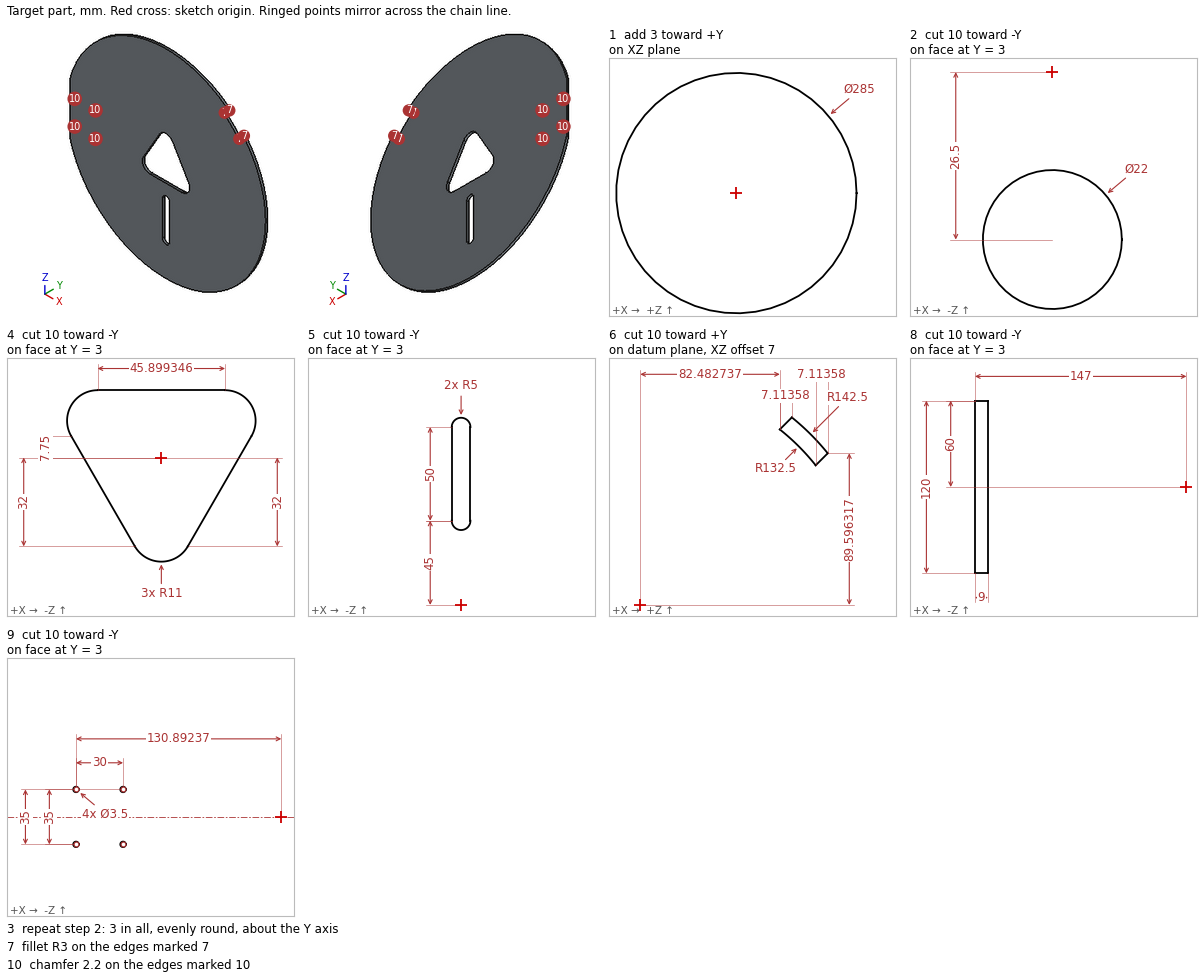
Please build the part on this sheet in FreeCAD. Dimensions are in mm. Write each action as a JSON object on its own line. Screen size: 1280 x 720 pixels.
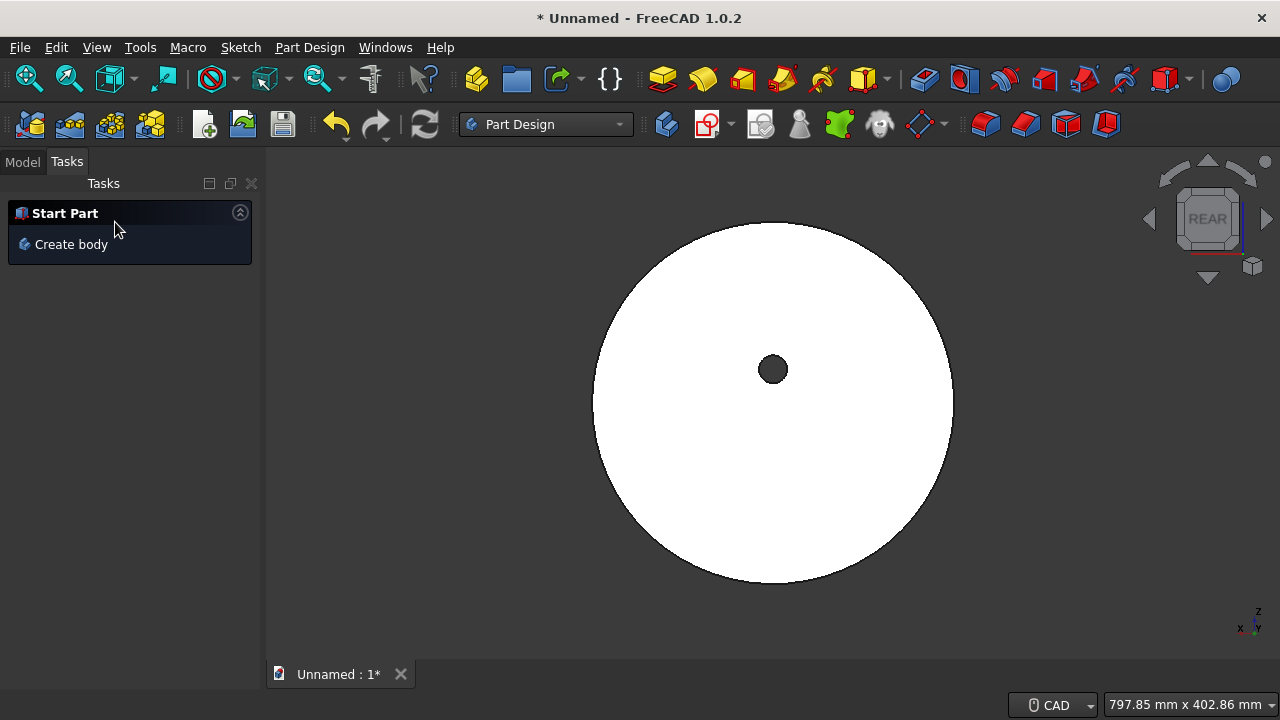
{"action": "left_click", "coordinate": [23, 161]}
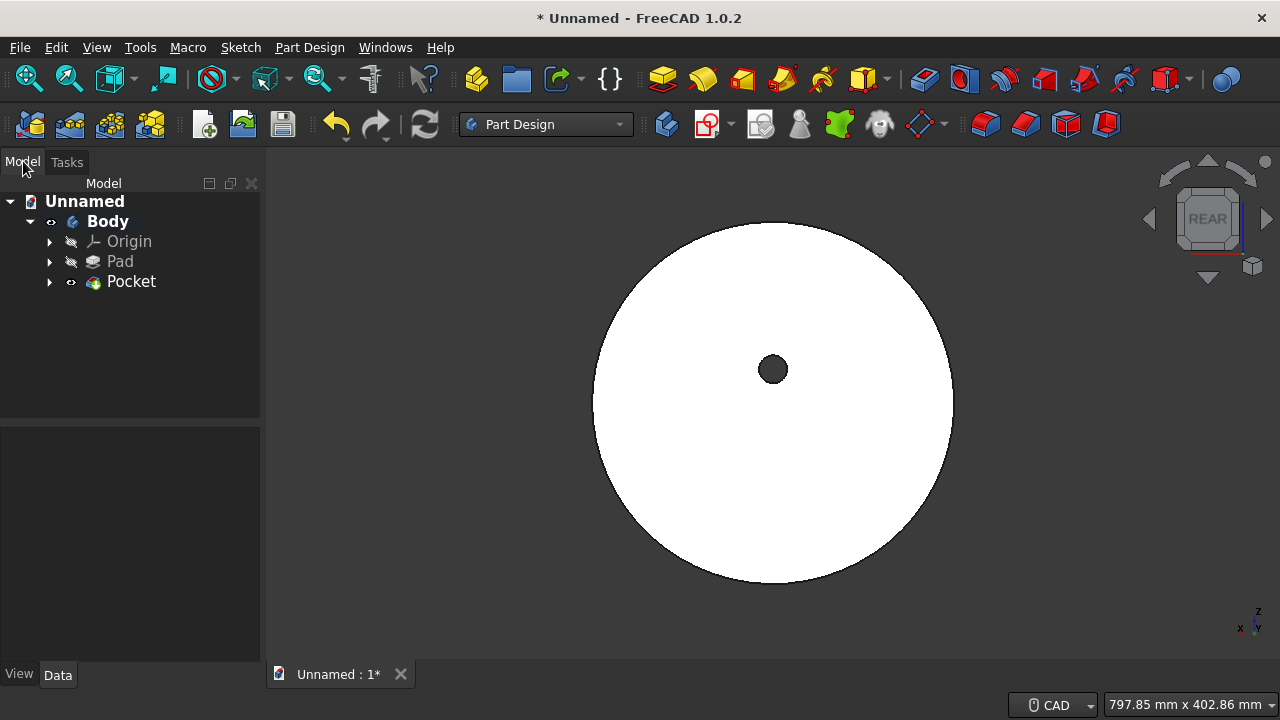
{"action": "left_click", "coordinate": [116, 282]}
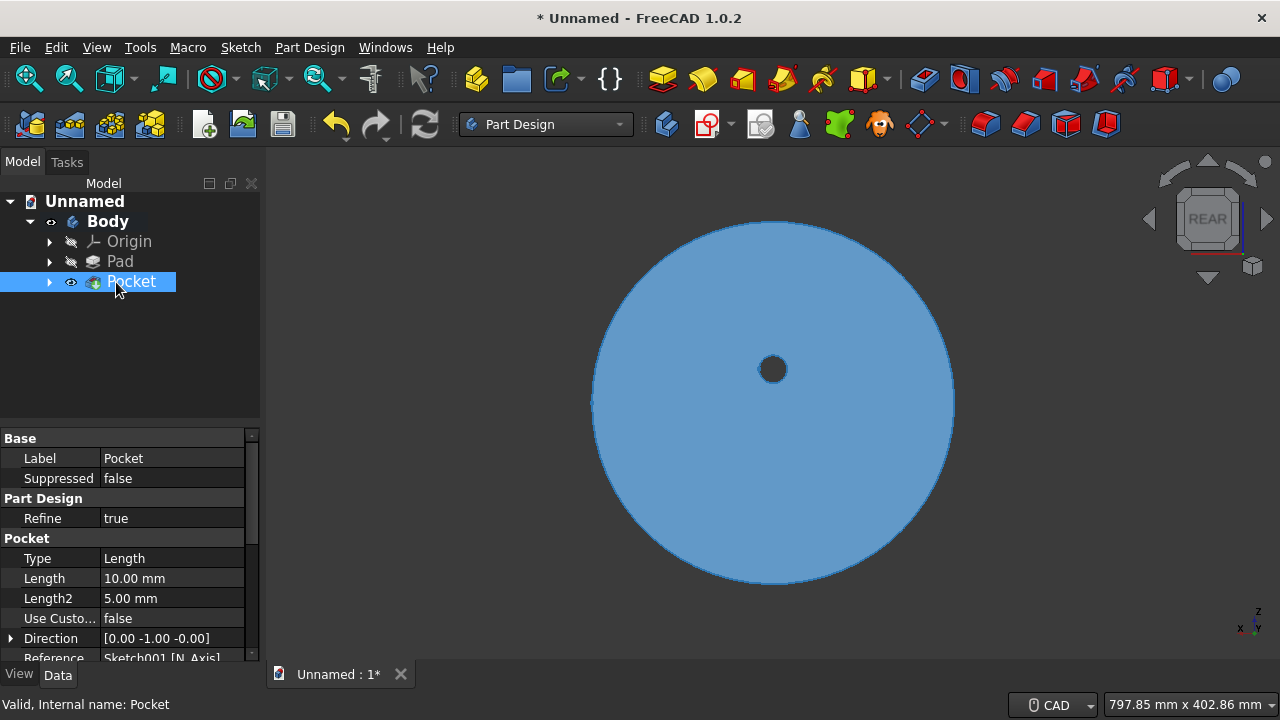
{"action": "left_click", "coordinate": [110, 124]}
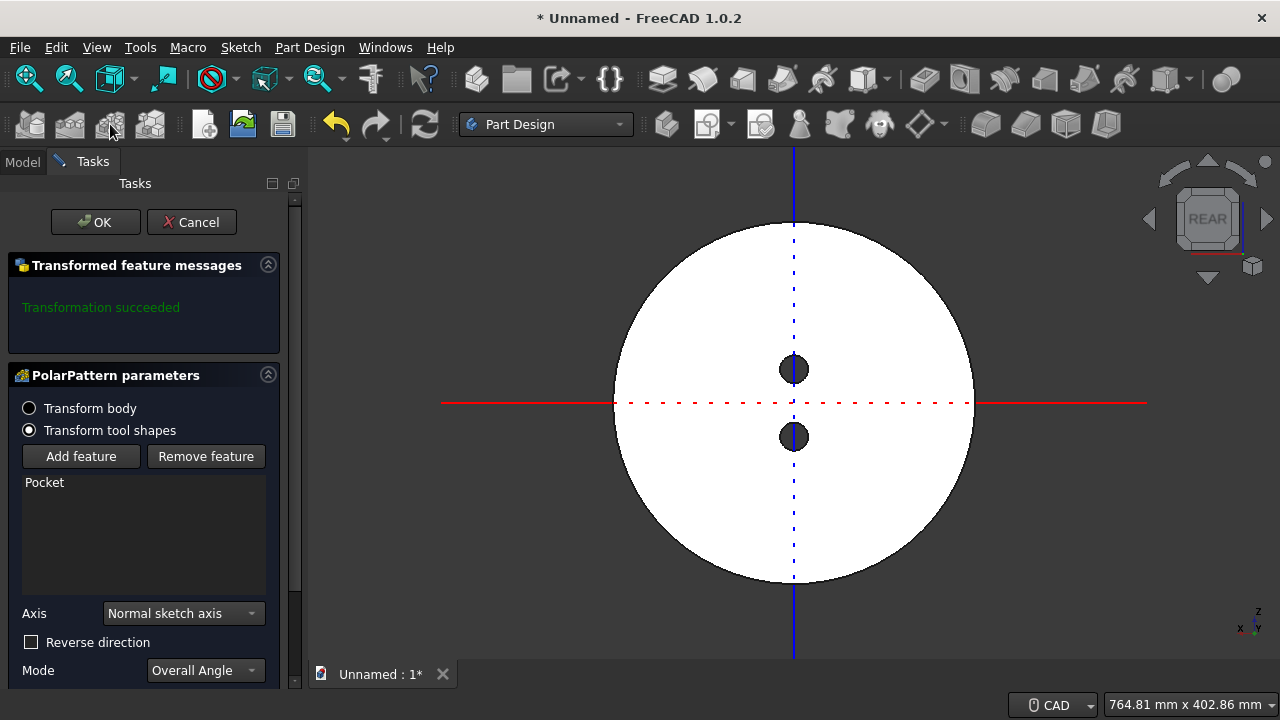
{"action": "left_click", "coordinate": [184, 614]}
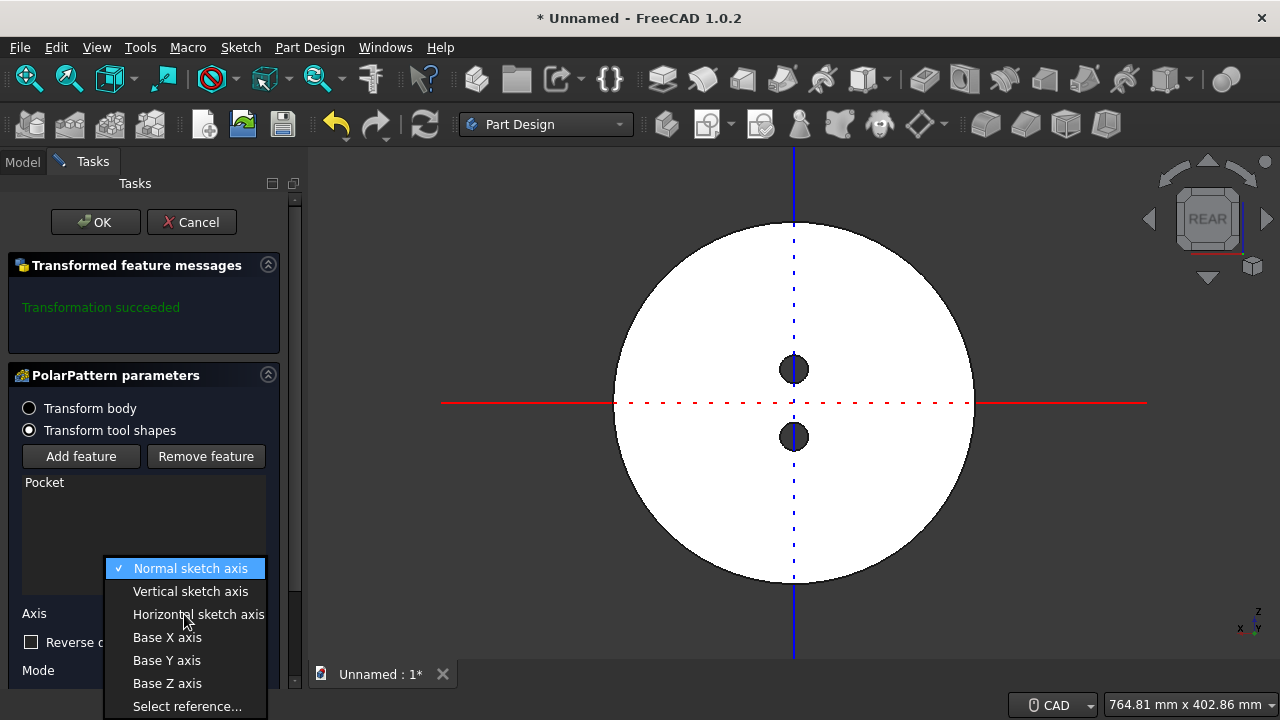
{"action": "left_click", "coordinate": [184, 660]}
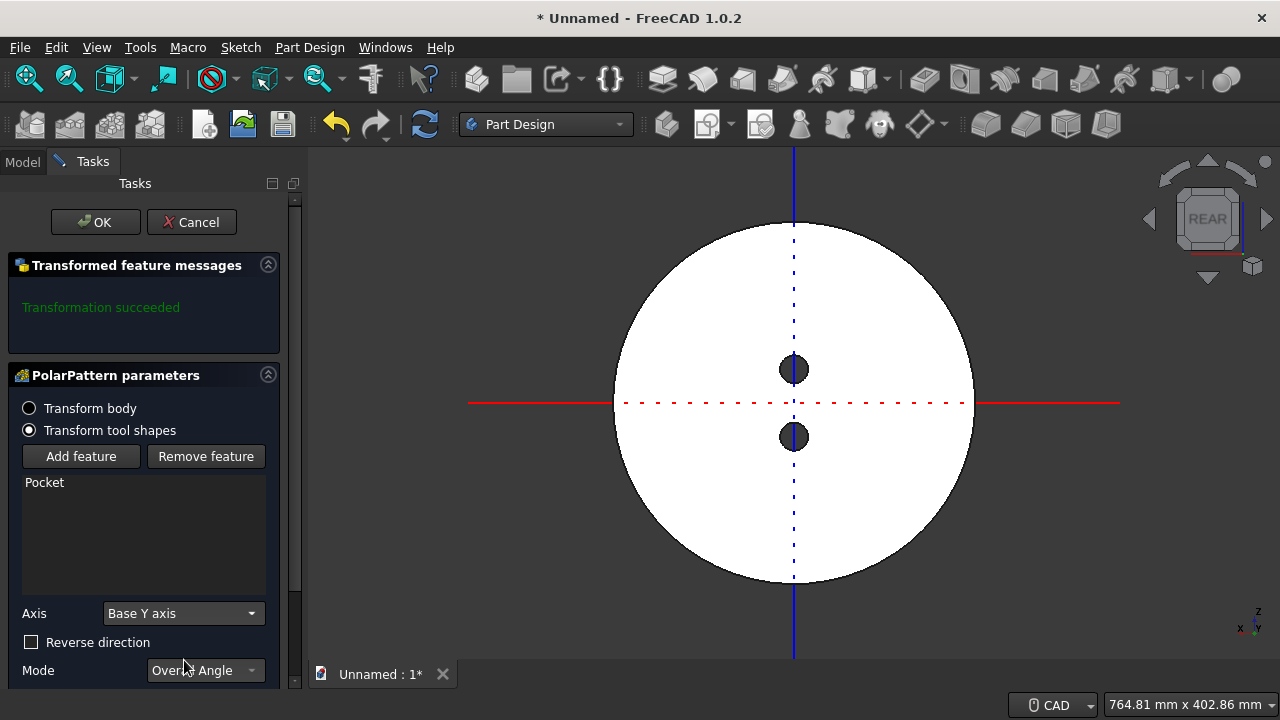
{"action": "scroll", "coordinate": [295, 440], "scroll_direction": "down", "scroll_amount": 2}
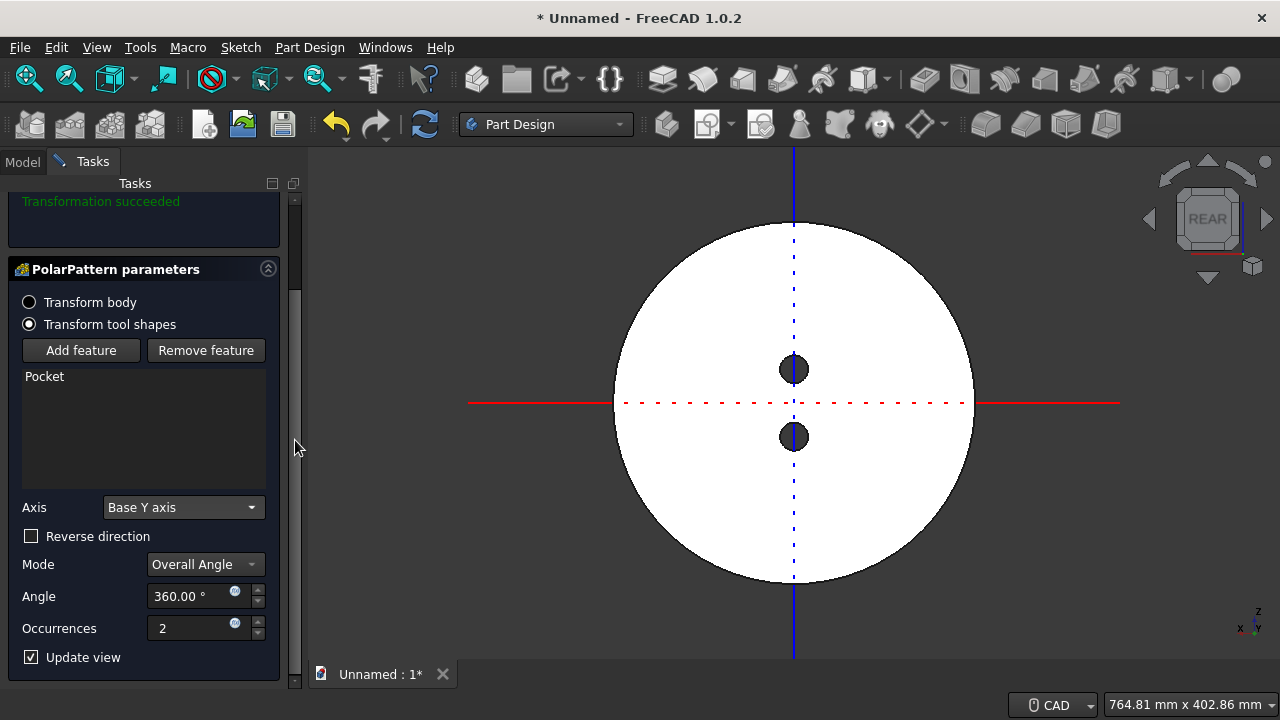
{"action": "triple_click", "coordinate": [198, 628]}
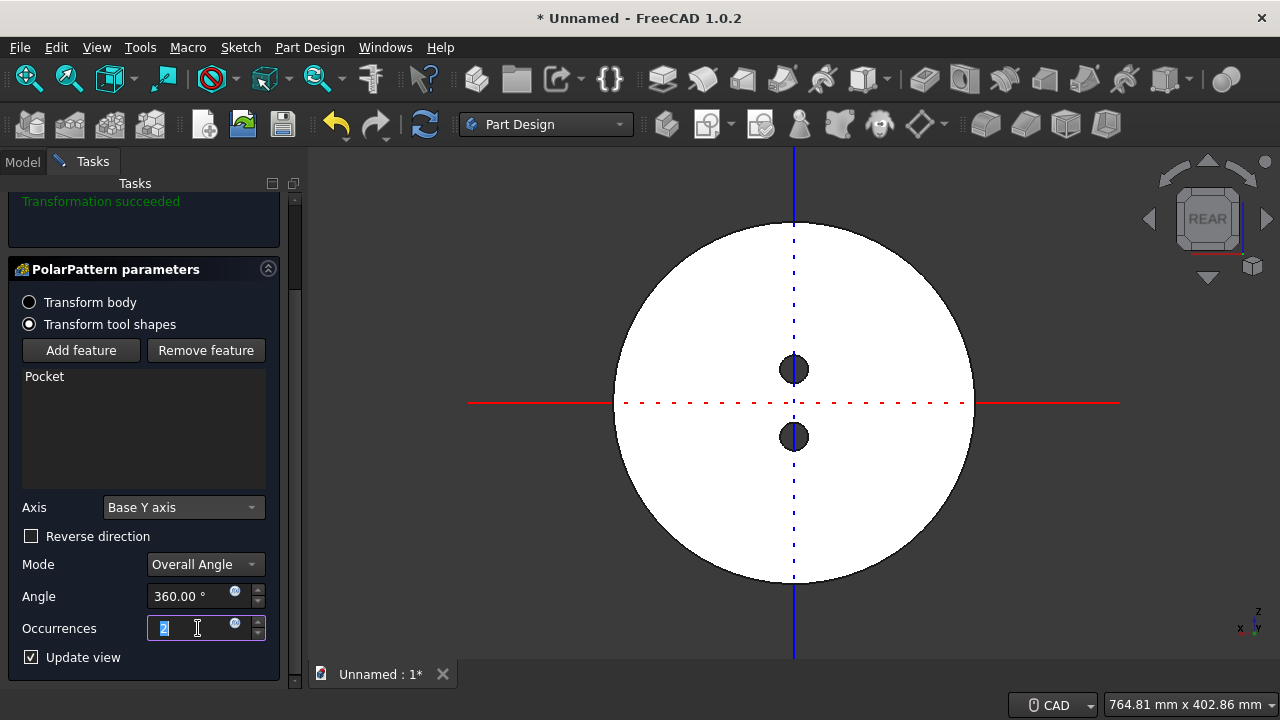
{"action": "type", "text": "3"}
{"action": "key", "text": "Tab"}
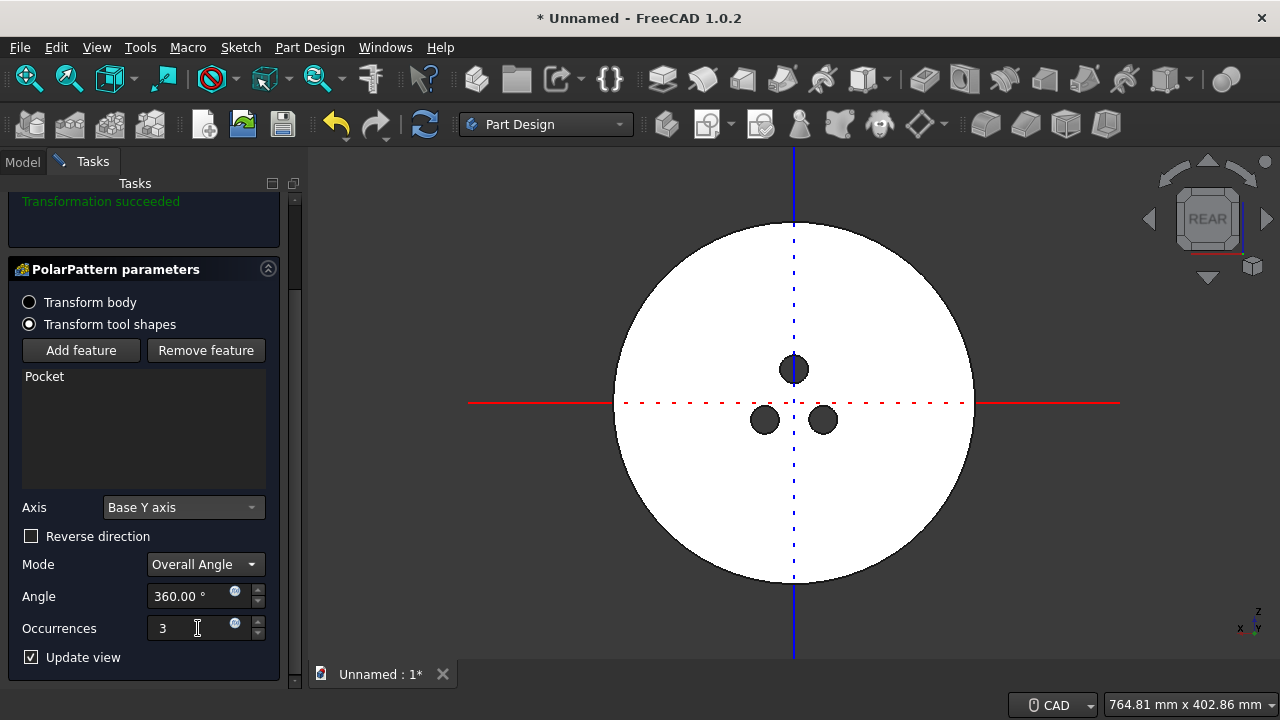
{"action": "scroll", "coordinate": [295, 440], "scroll_direction": "up", "scroll_amount": 3}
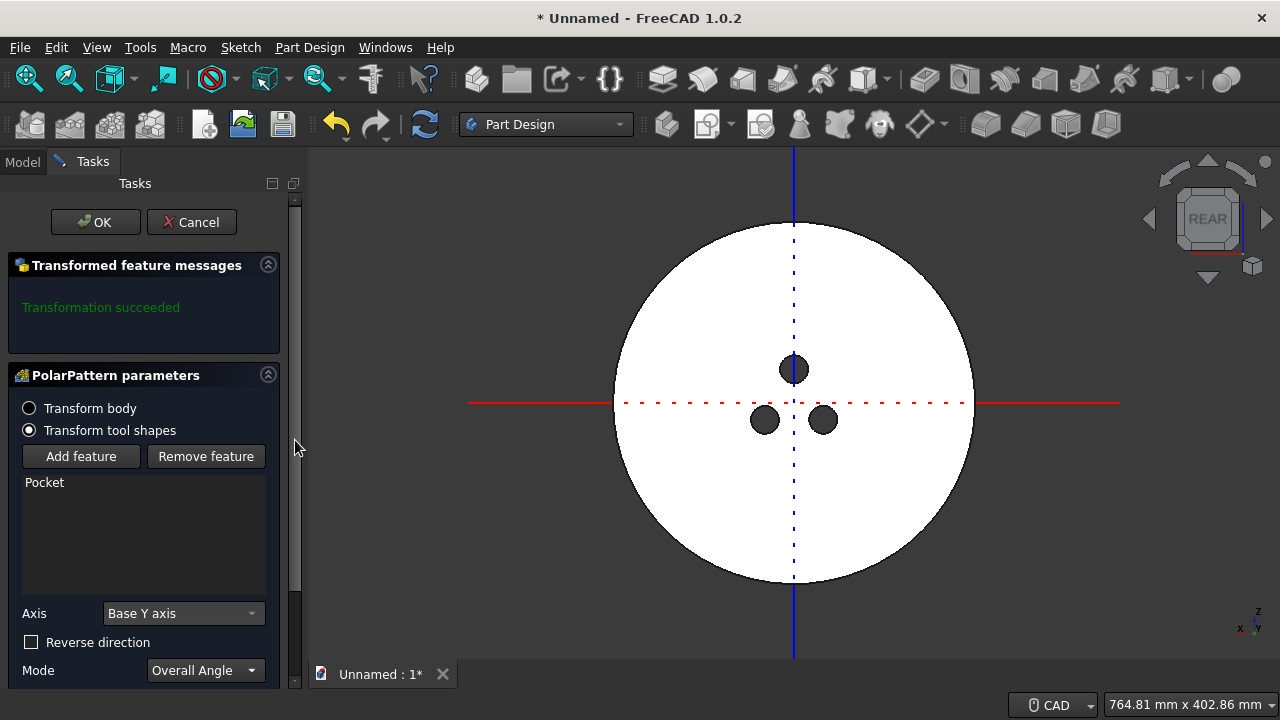
{"action": "left_click", "coordinate": [96, 222]}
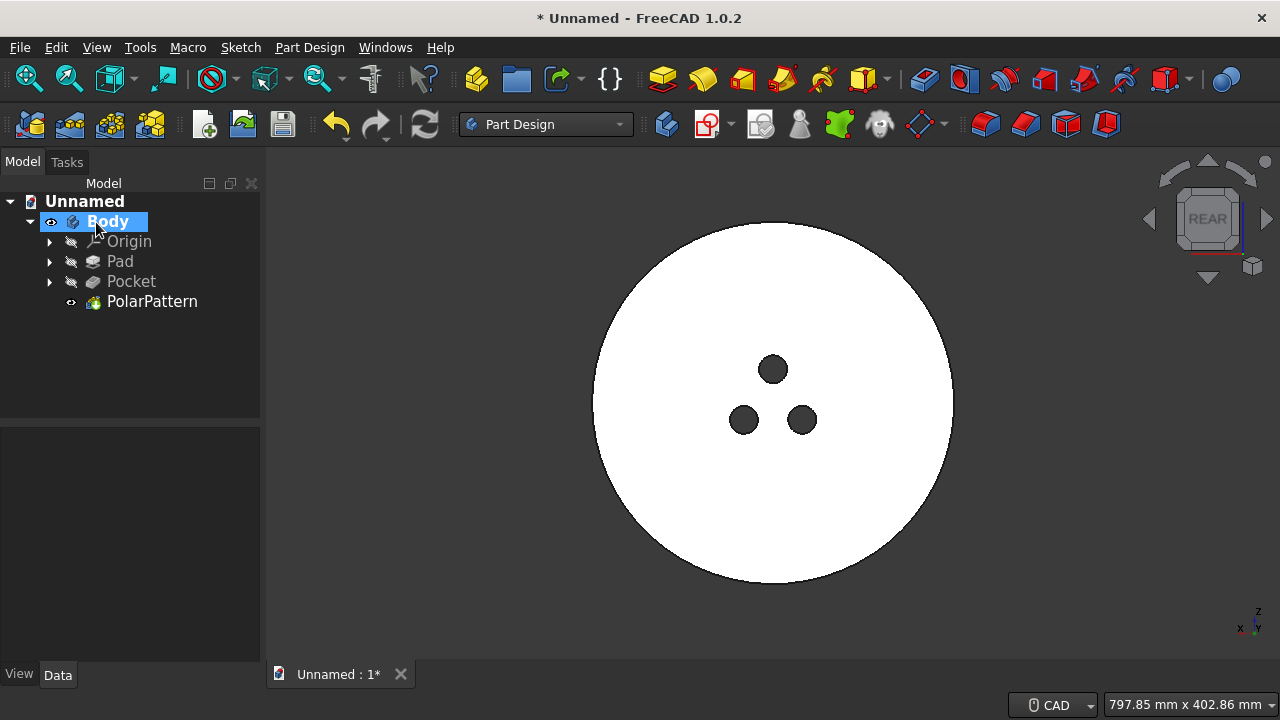
{"action": "left_click", "coordinate": [773, 505]}